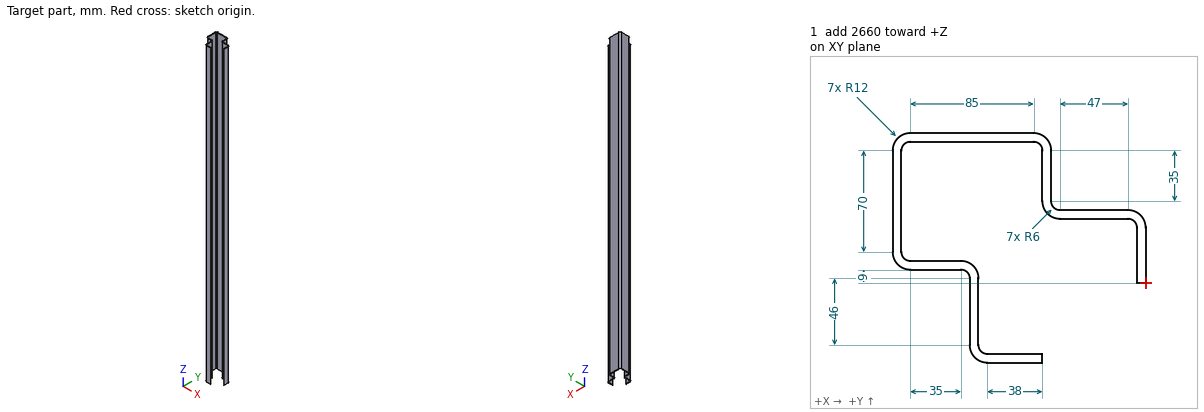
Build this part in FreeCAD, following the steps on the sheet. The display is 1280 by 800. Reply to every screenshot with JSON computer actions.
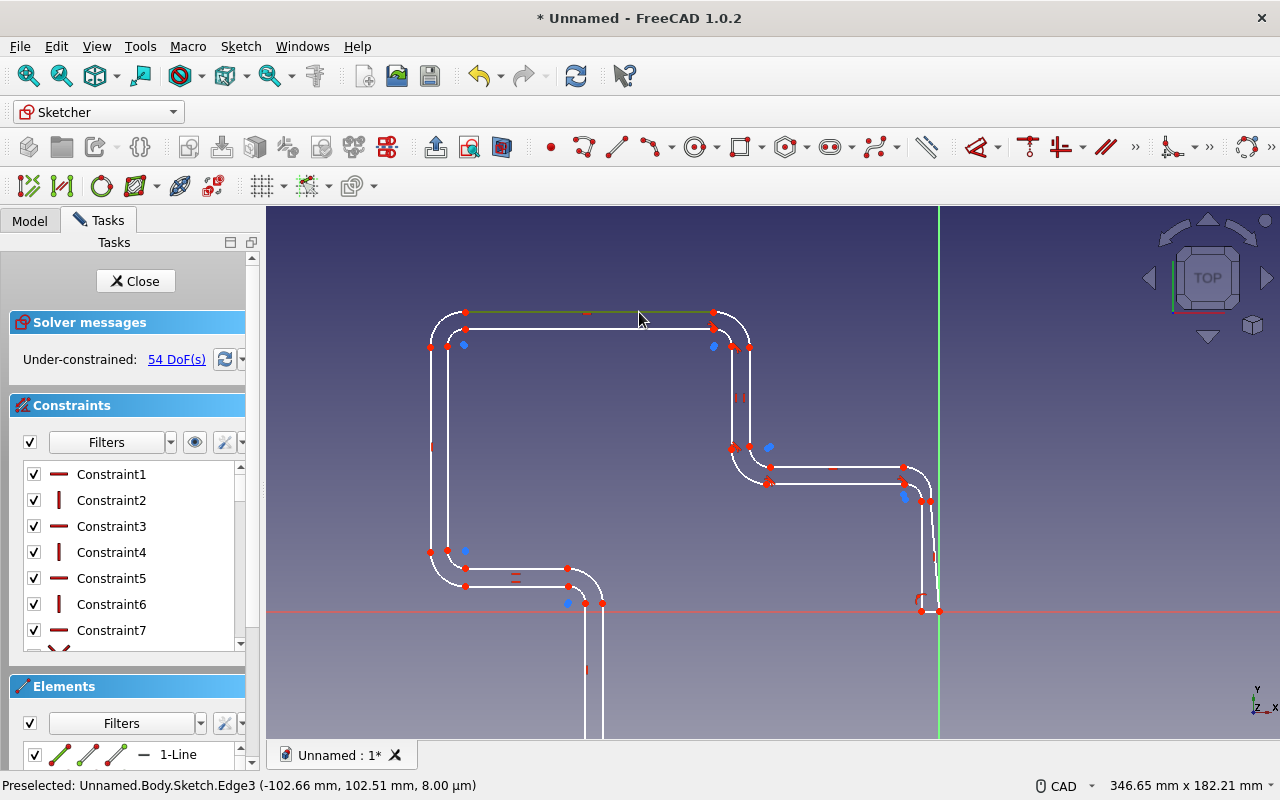
{"action": "left_click", "coordinate": [449, 315]}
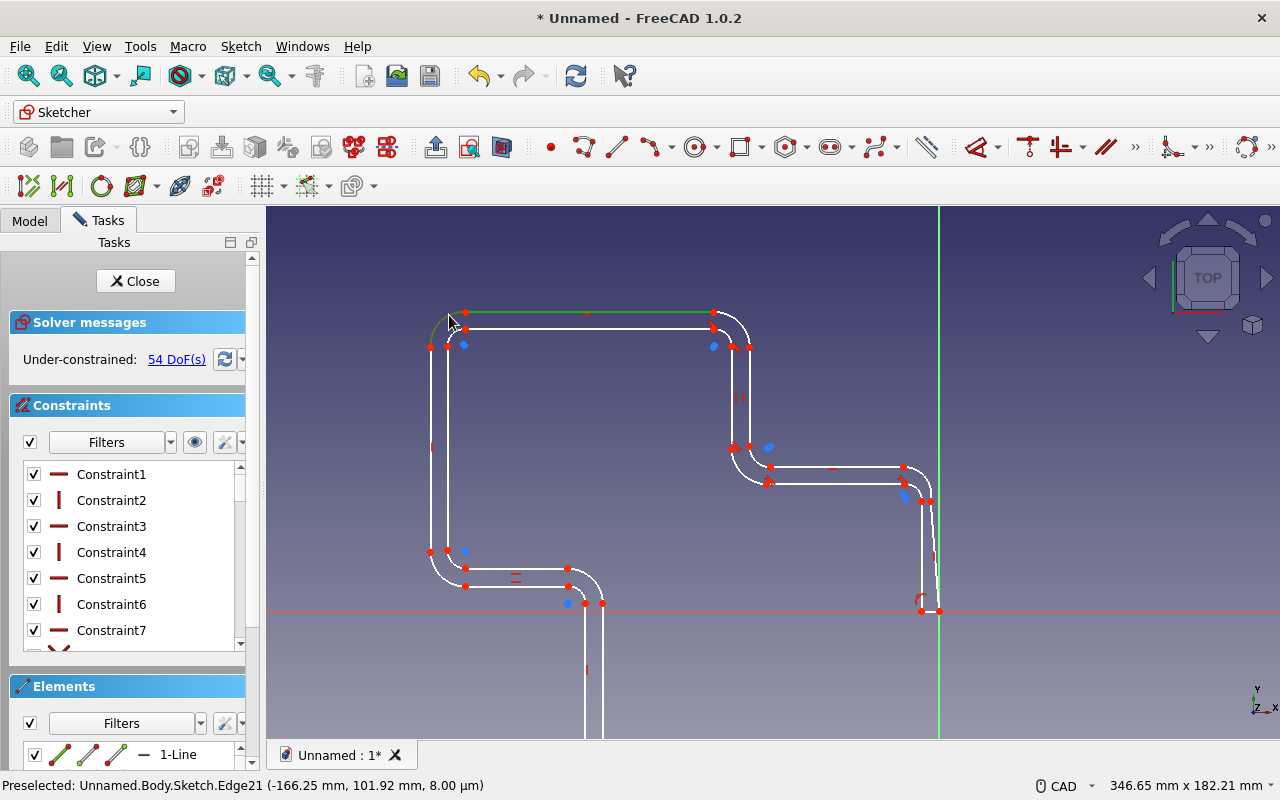
{"action": "key", "text": "t"}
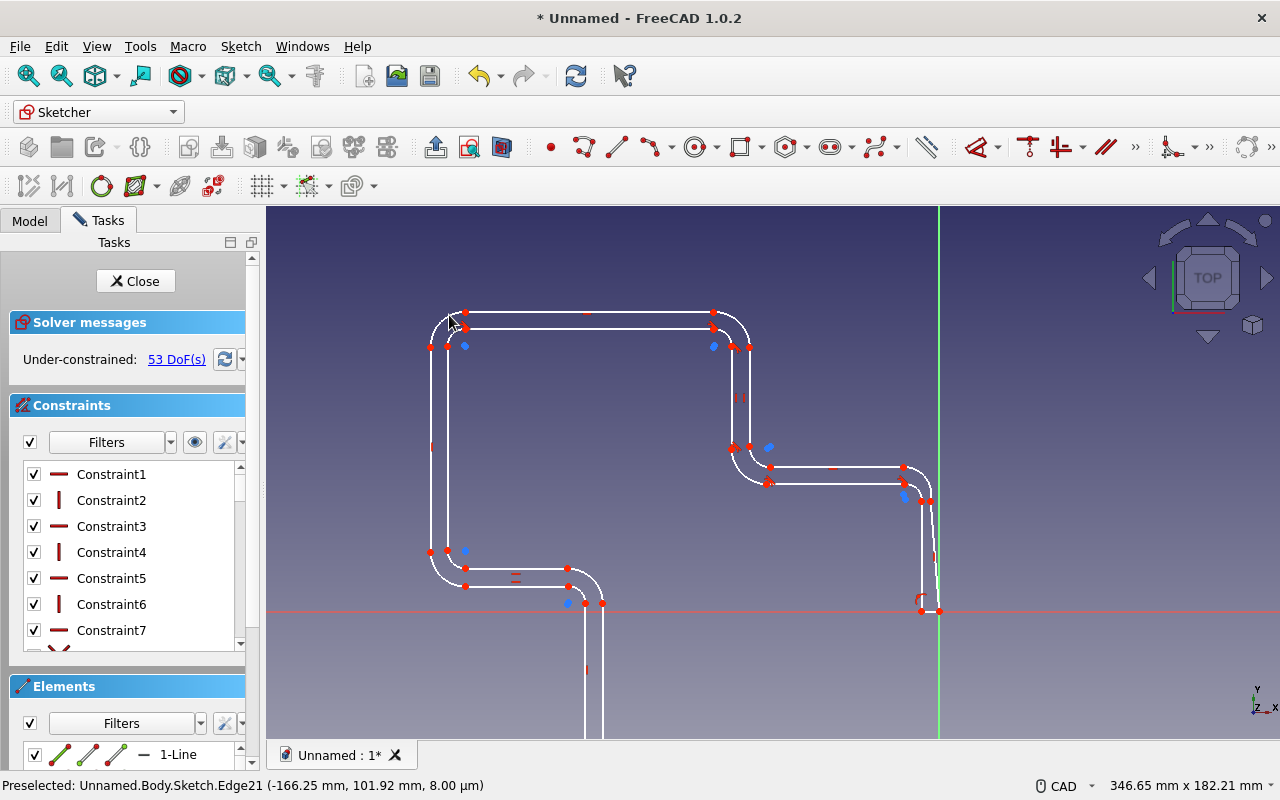
{"action": "left_click", "coordinate": [431, 409]}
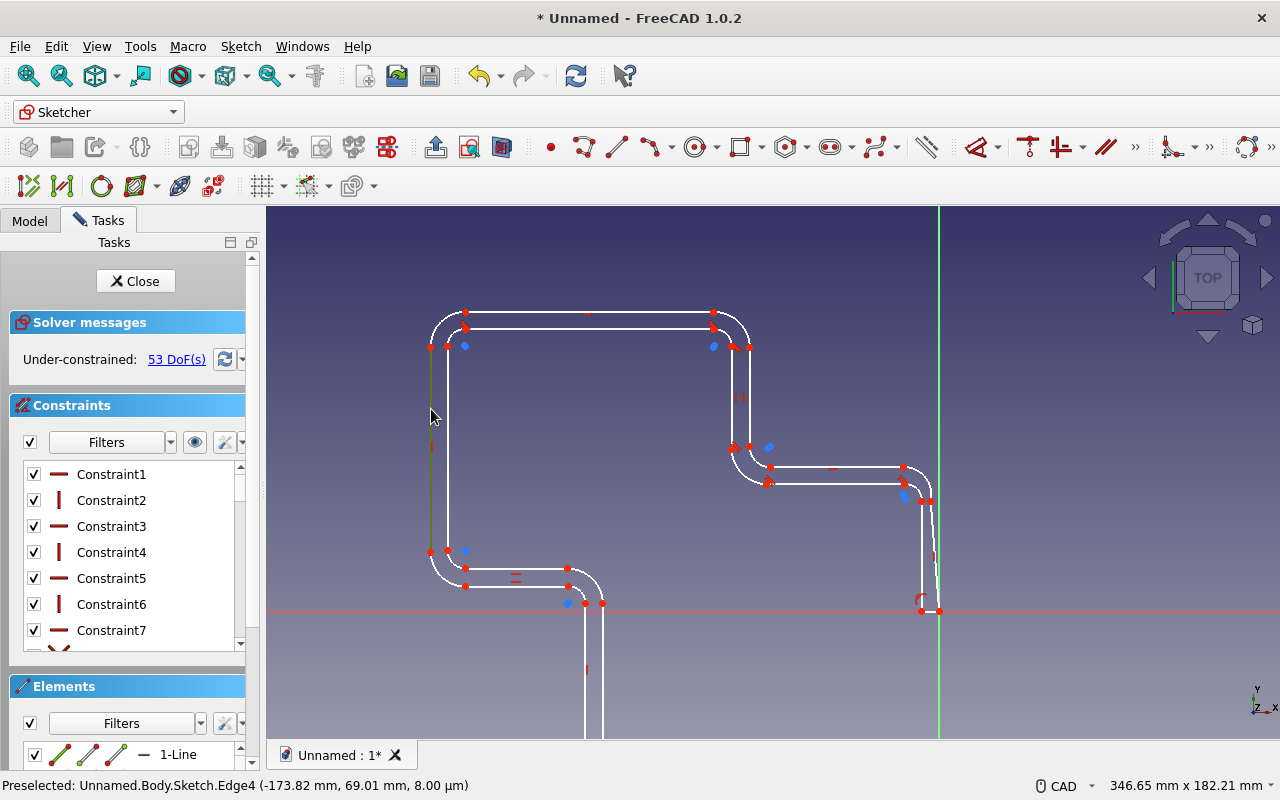
{"action": "left_click", "coordinate": [449, 316]}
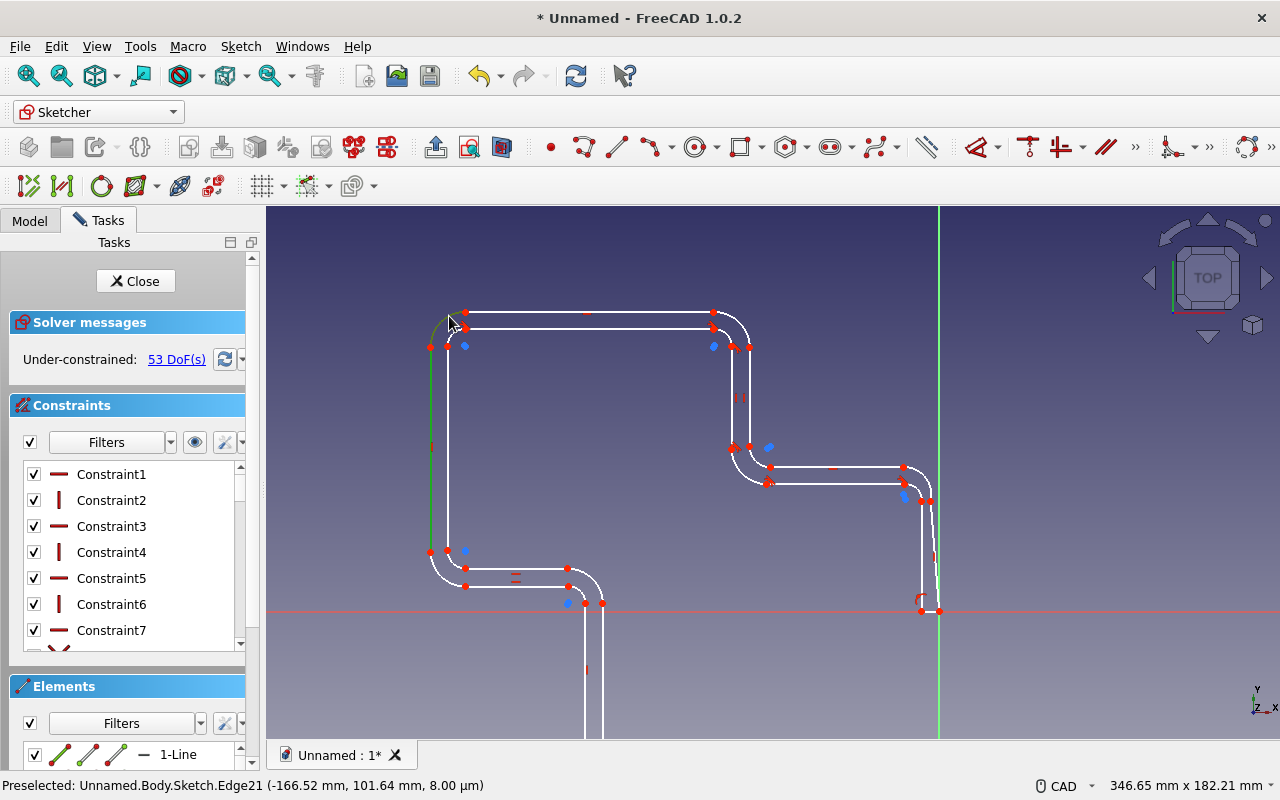
{"action": "key", "text": "t"}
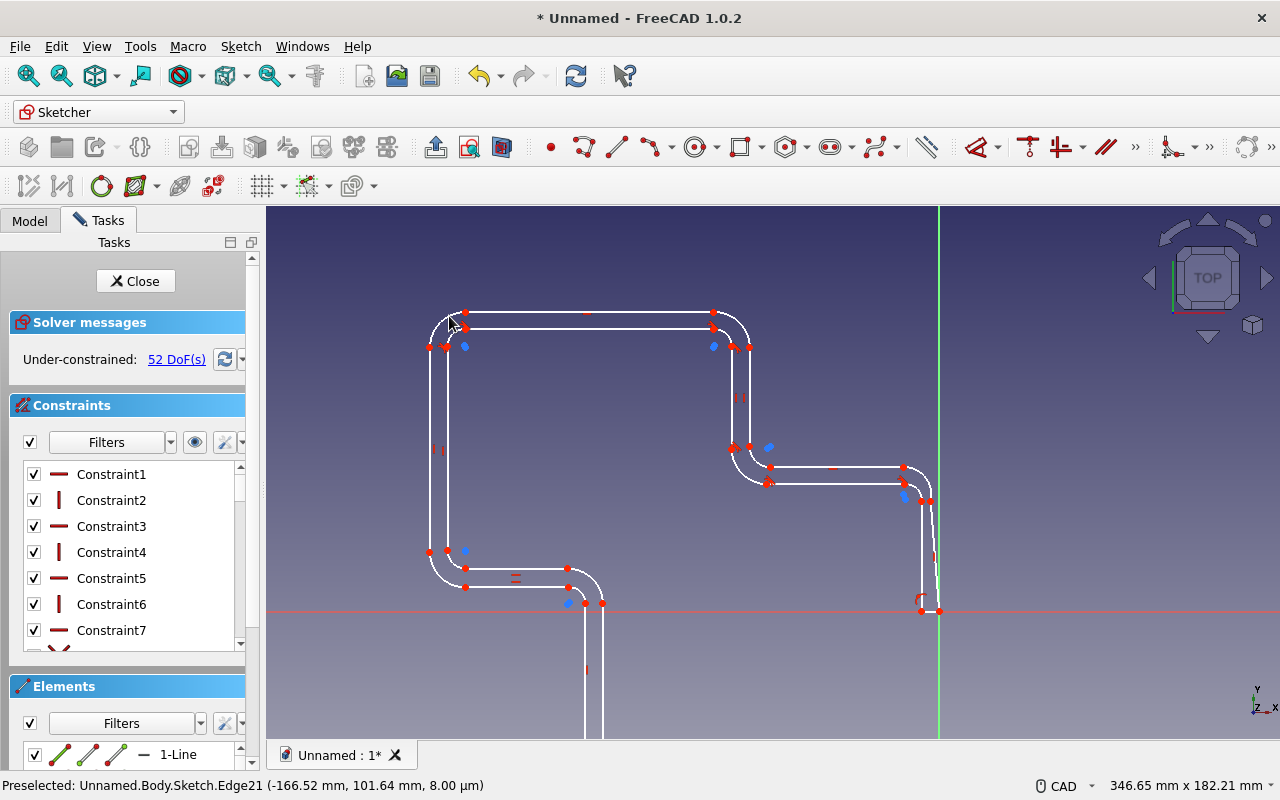
{"action": "left_click", "coordinate": [430, 409]}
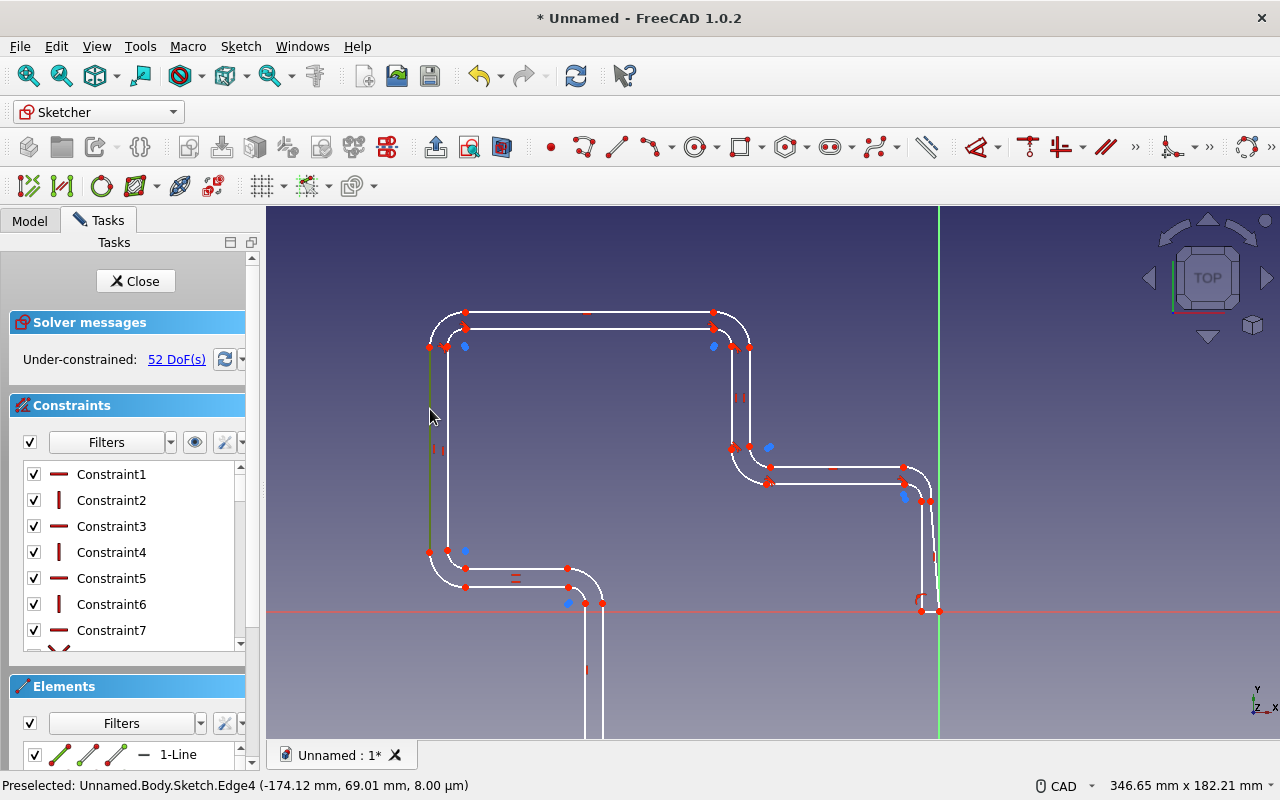
{"action": "left_click", "coordinate": [434, 568]}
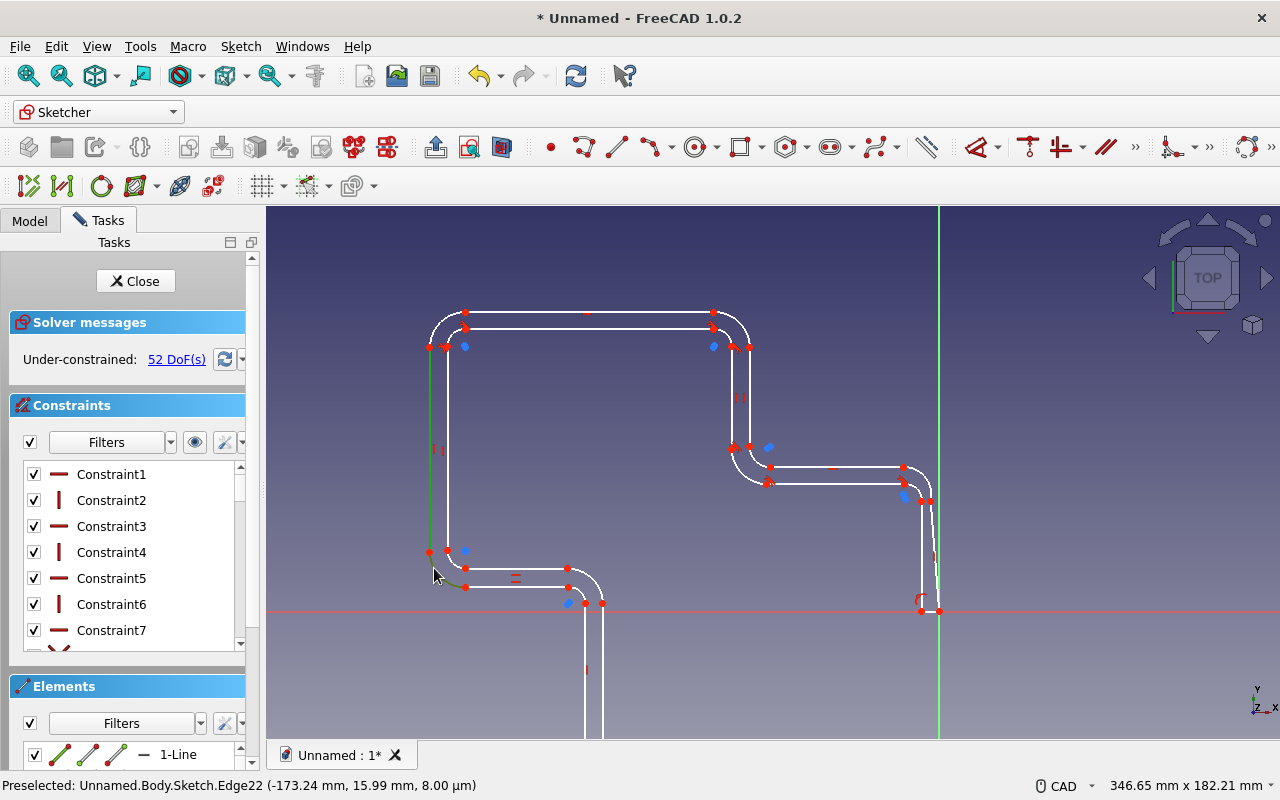
{"action": "key", "text": "t"}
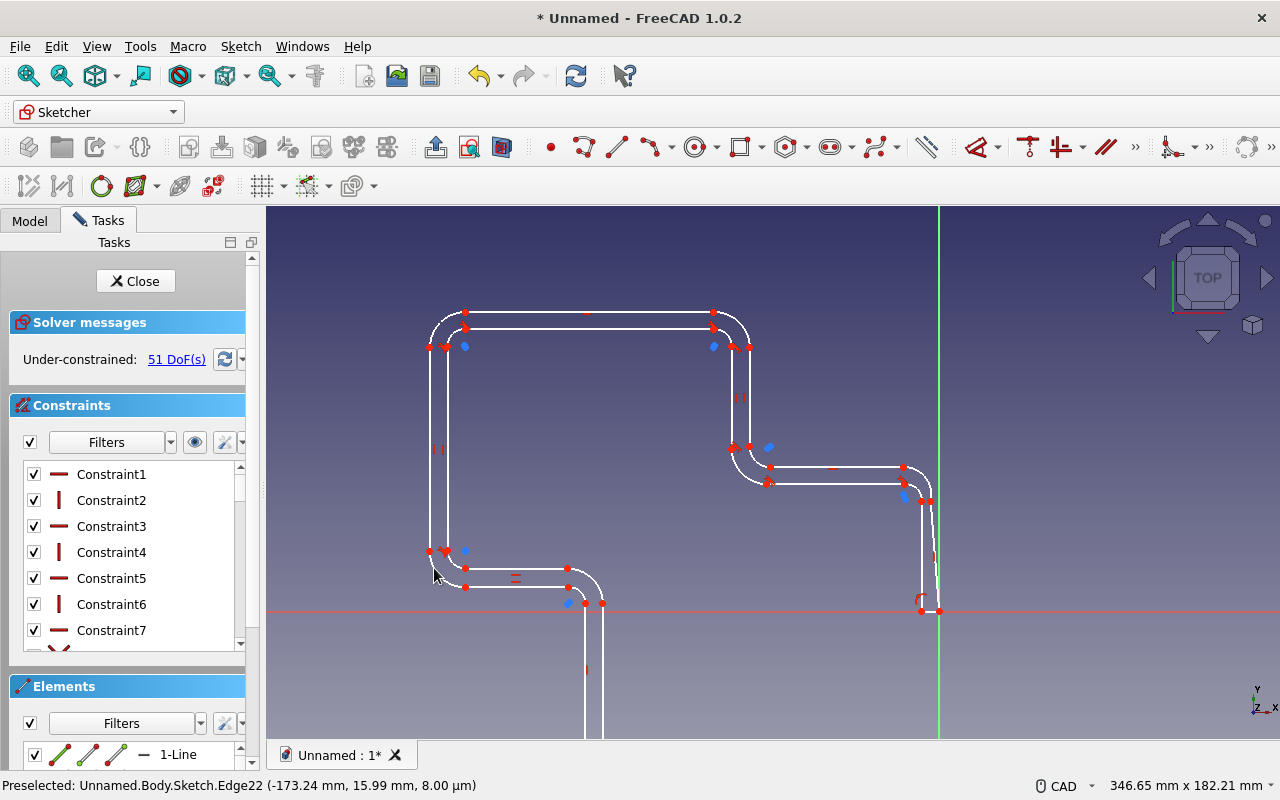
{"action": "left_click", "coordinate": [496, 587]}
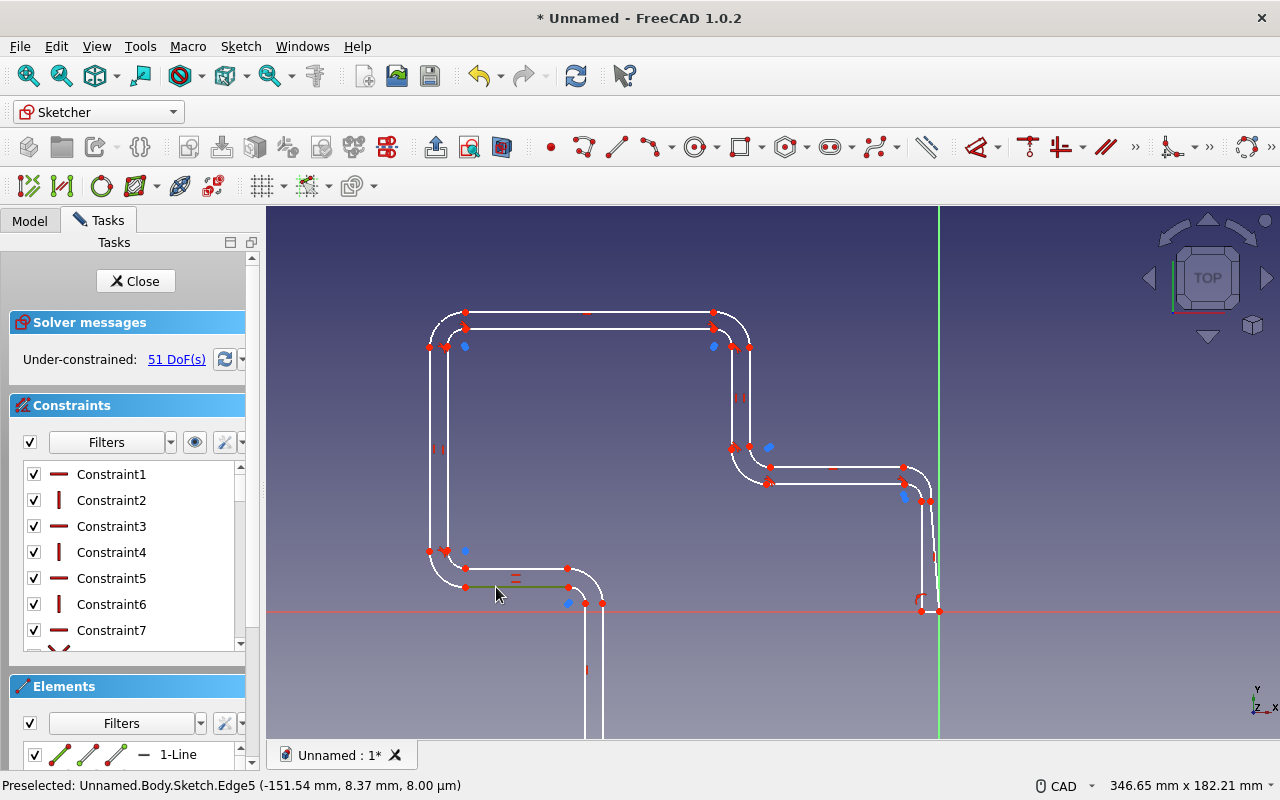
{"action": "left_click", "coordinate": [434, 568]}